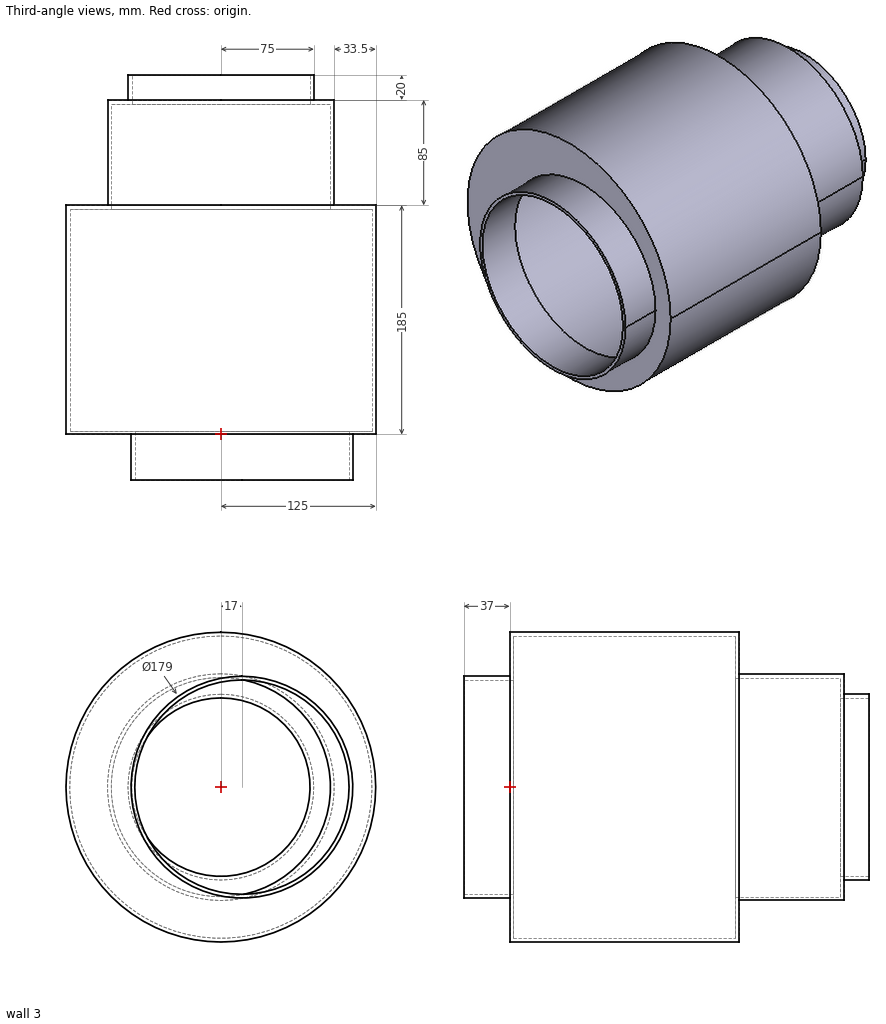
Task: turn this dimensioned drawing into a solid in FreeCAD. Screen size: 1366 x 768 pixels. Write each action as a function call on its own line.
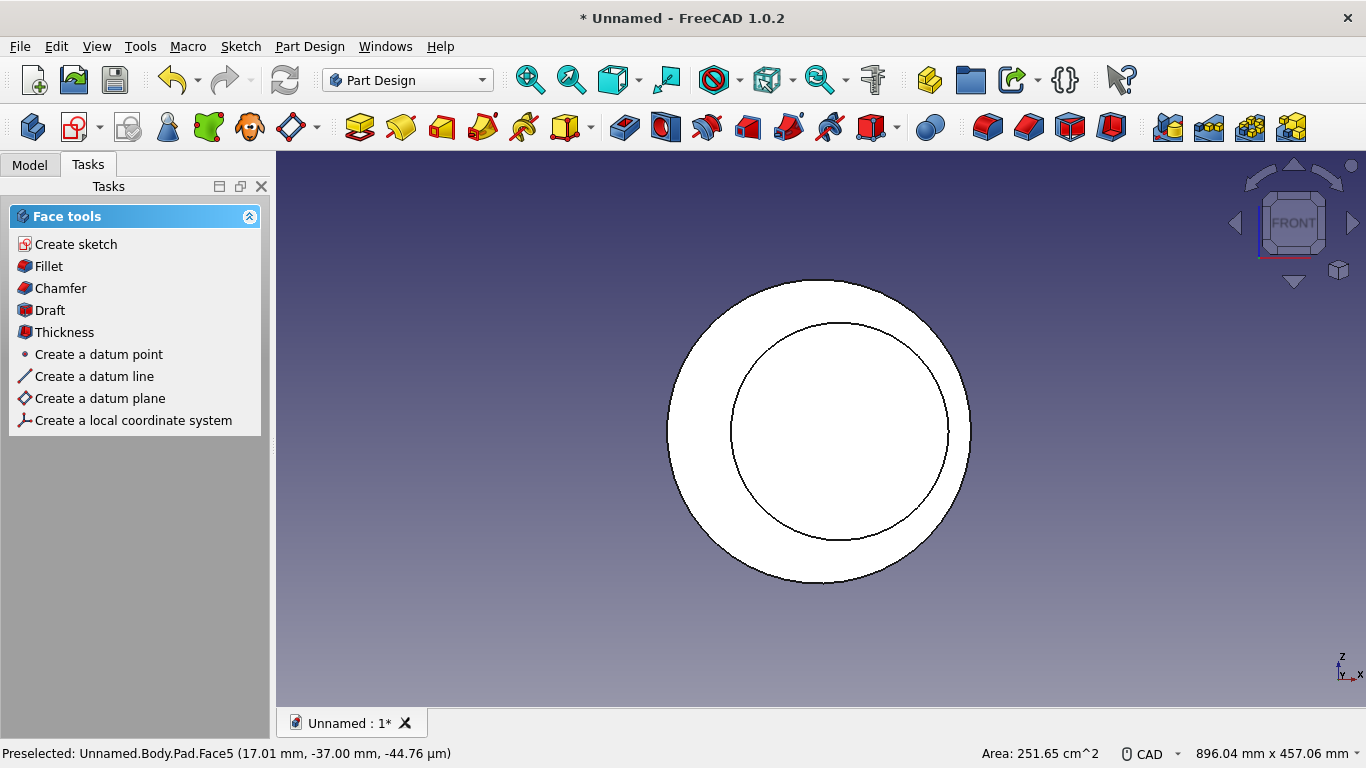
key(3)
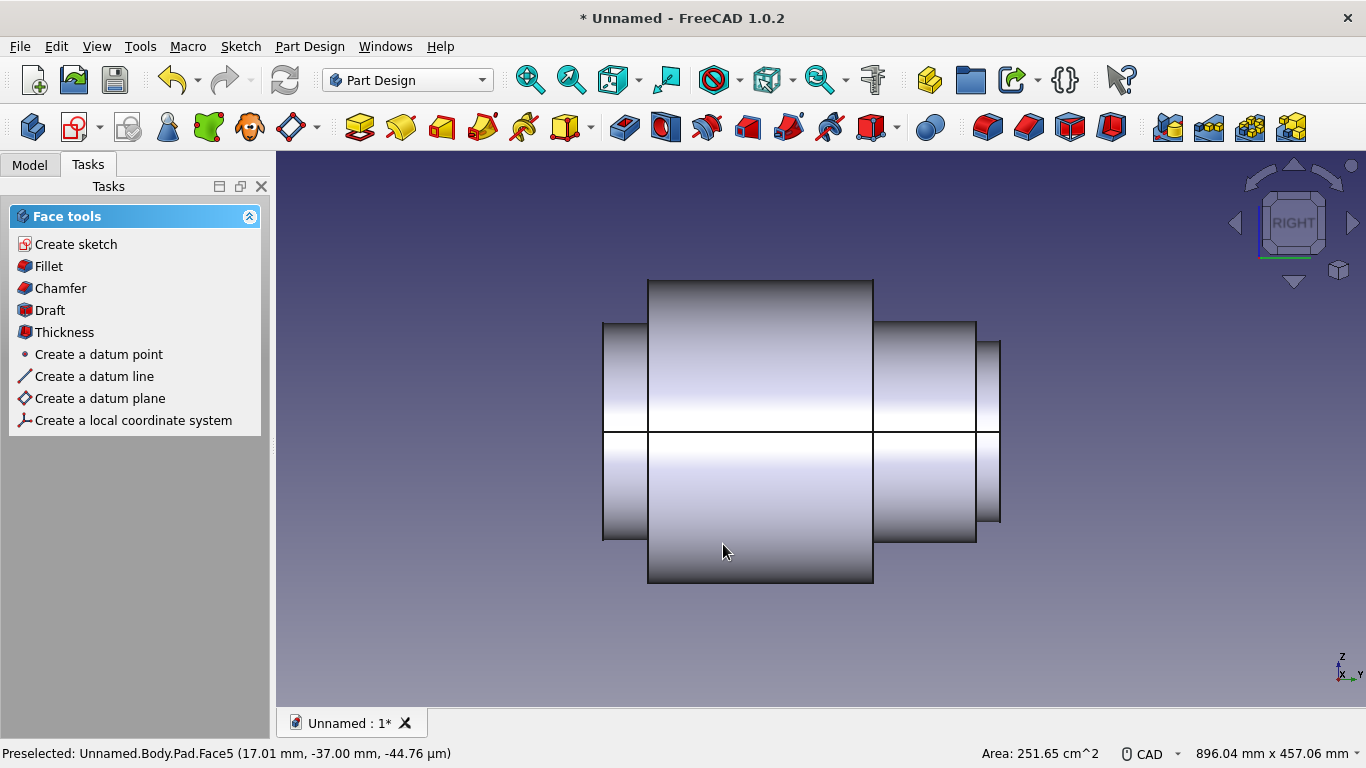
key(5)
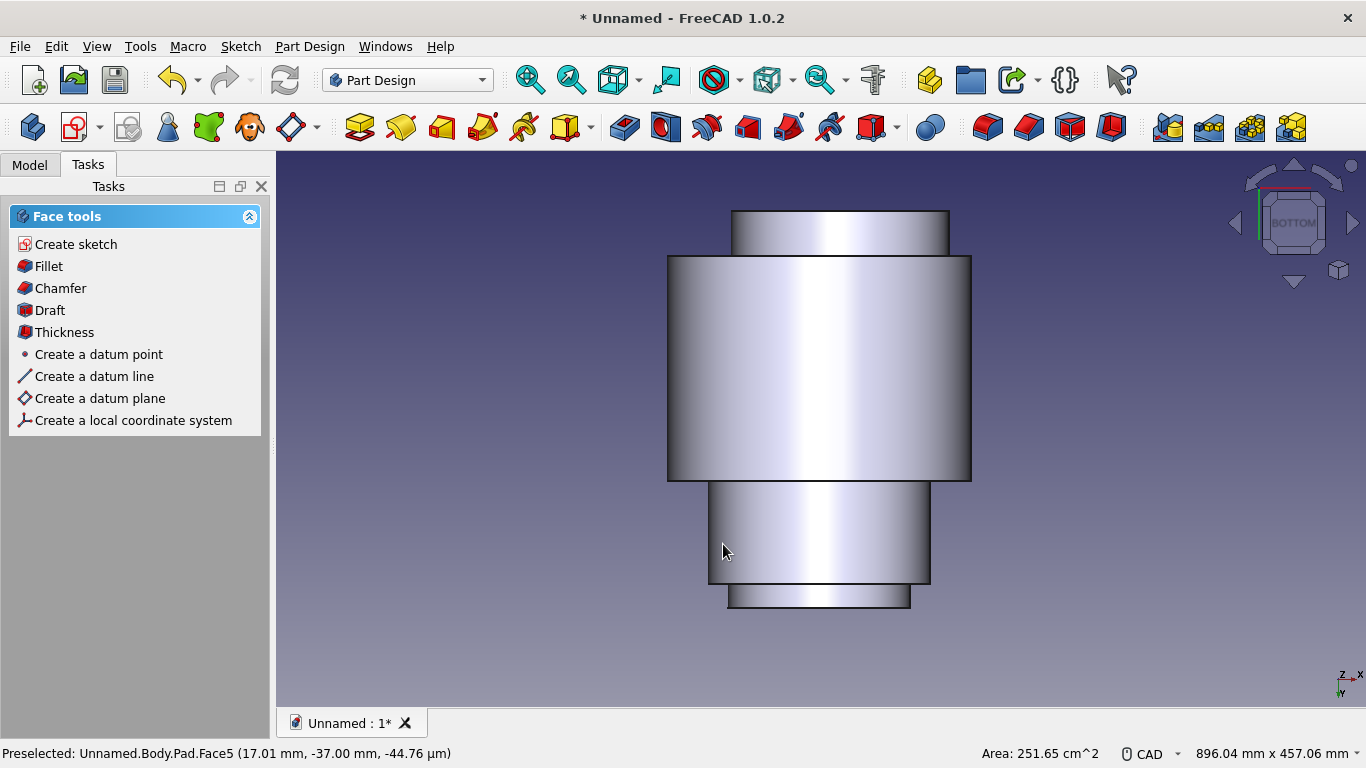
key(4)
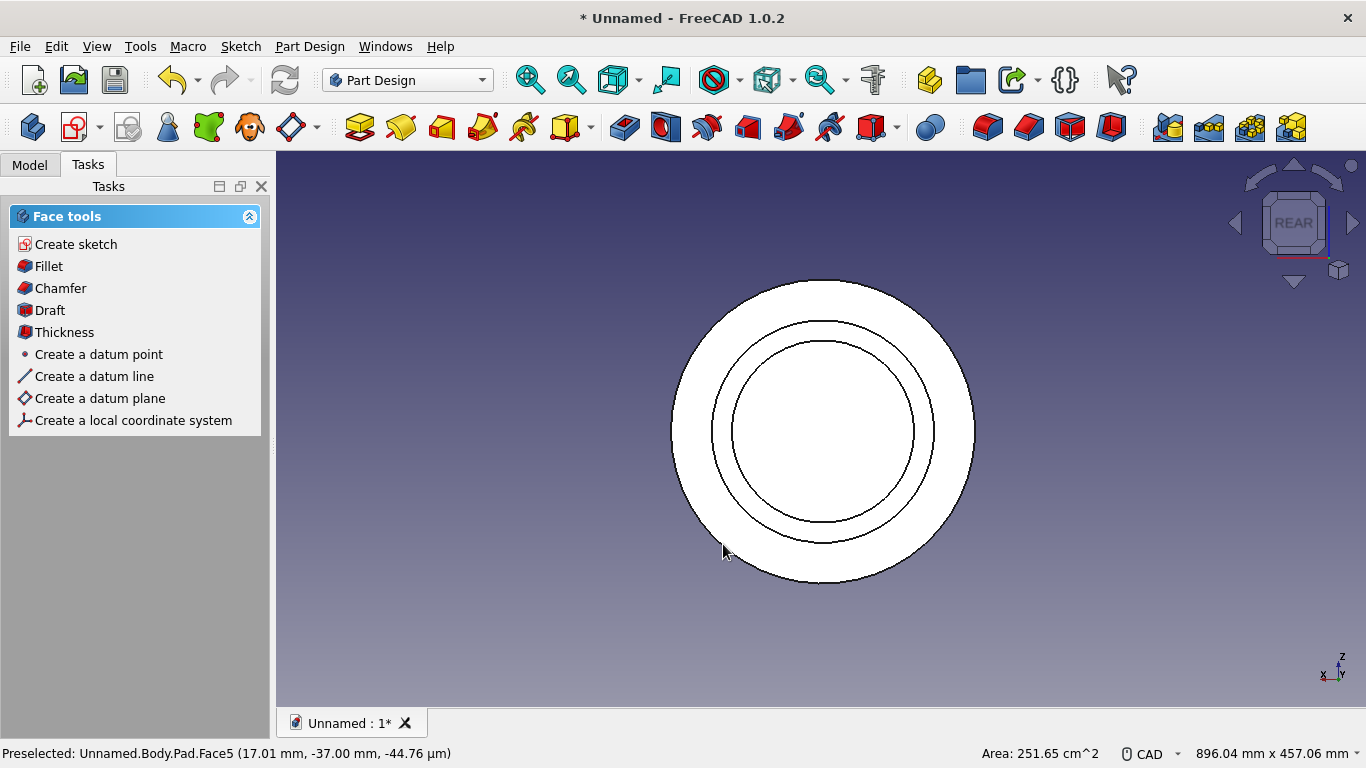
click(823, 431, ctrl)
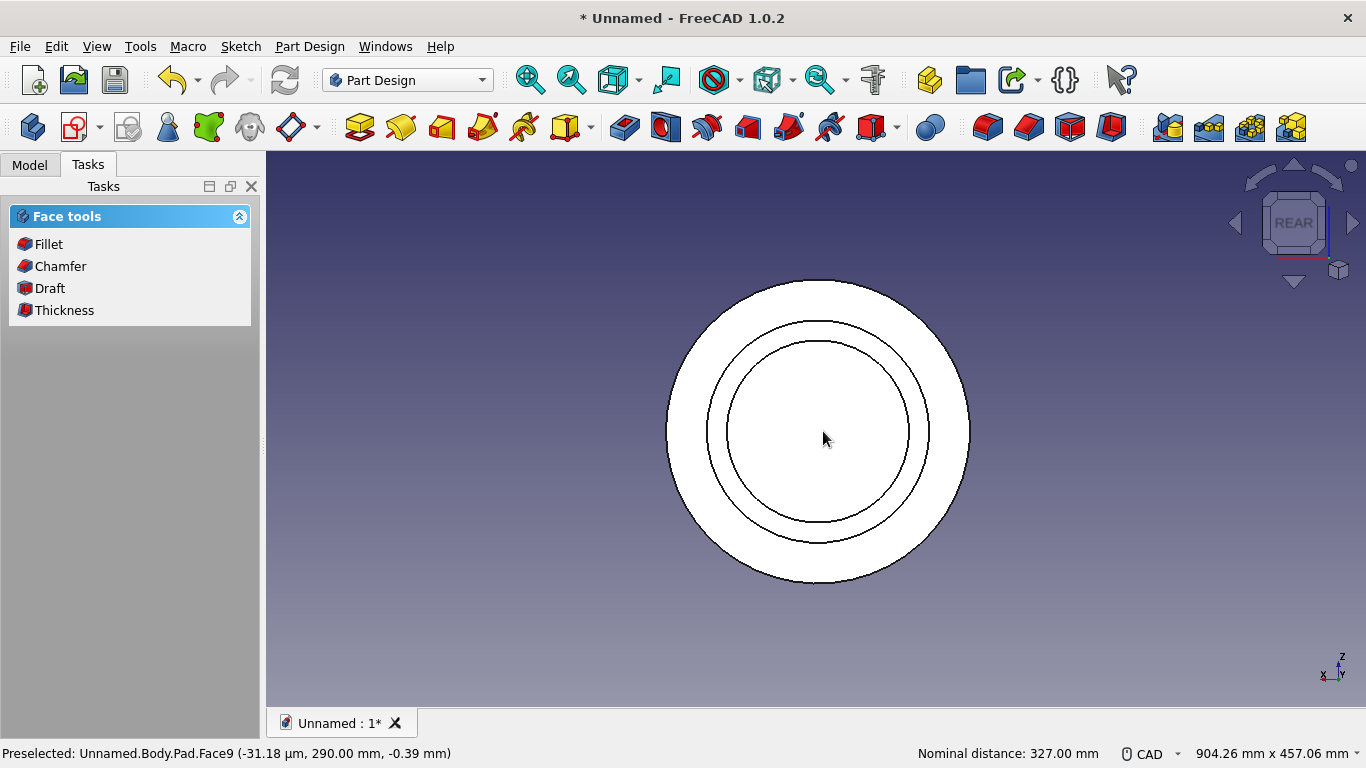
click(1111, 128)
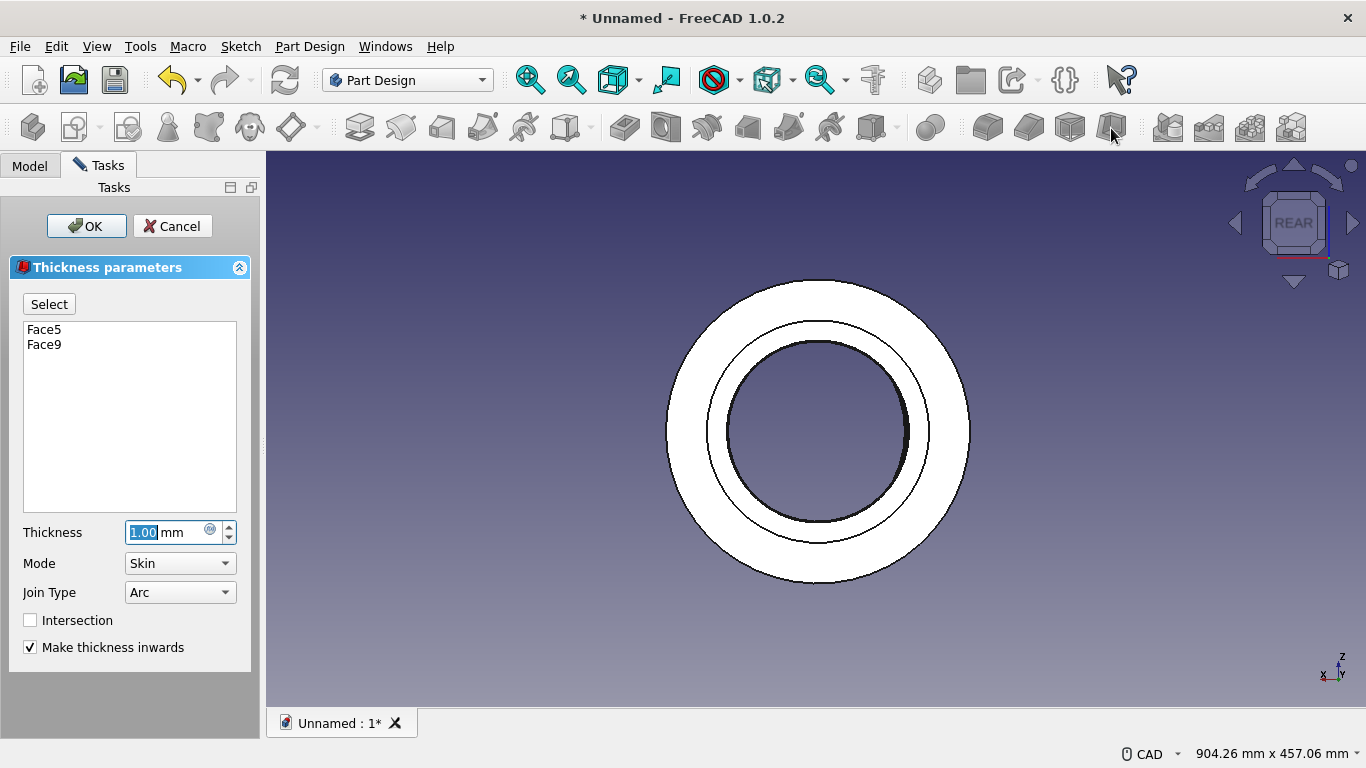
text(3)
key(Tab)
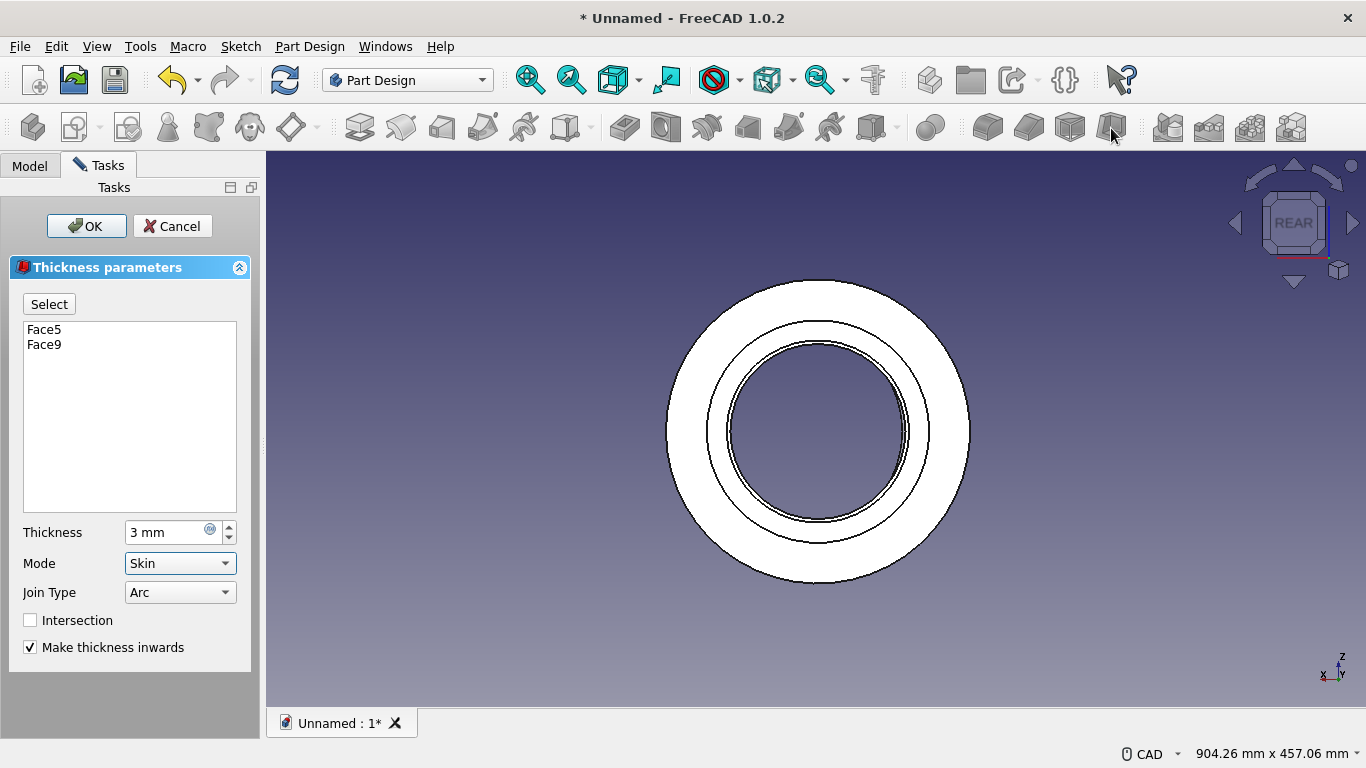
click(181, 592)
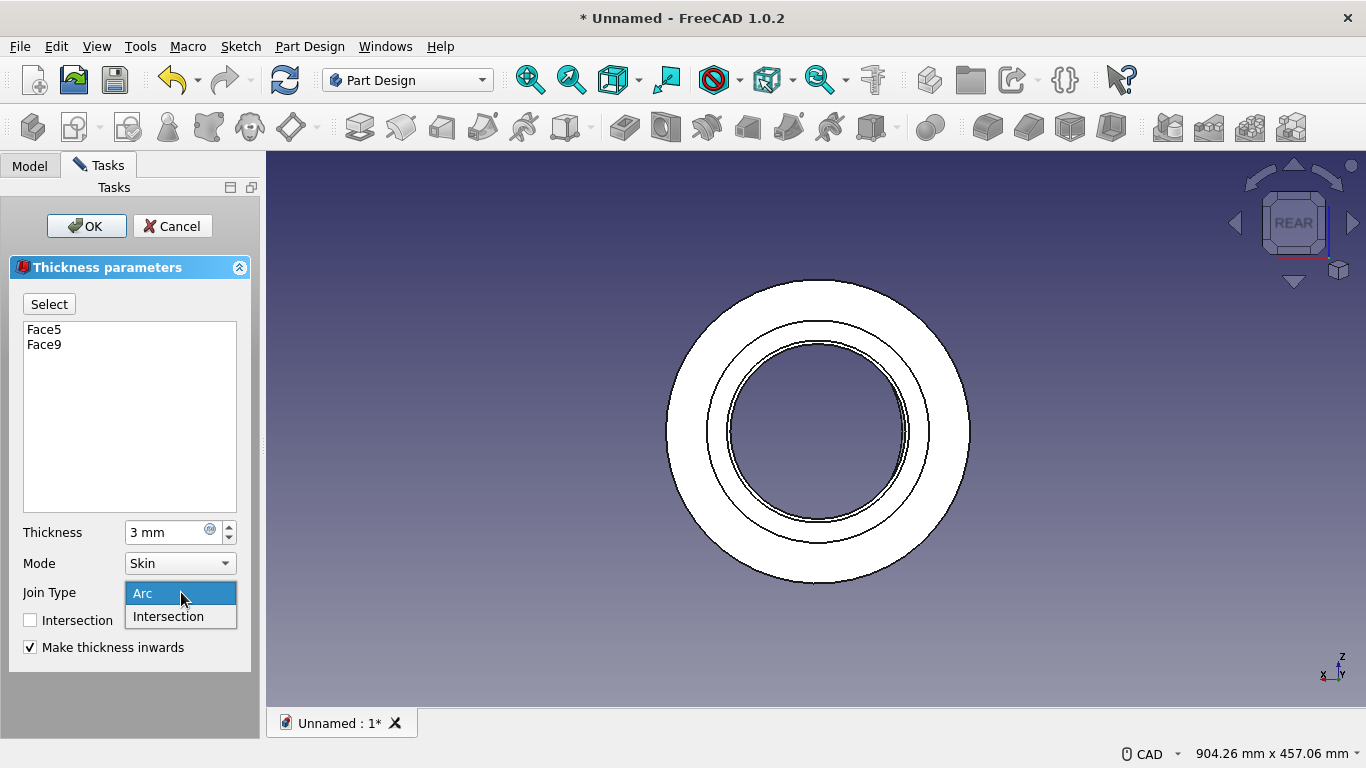
click(179, 616)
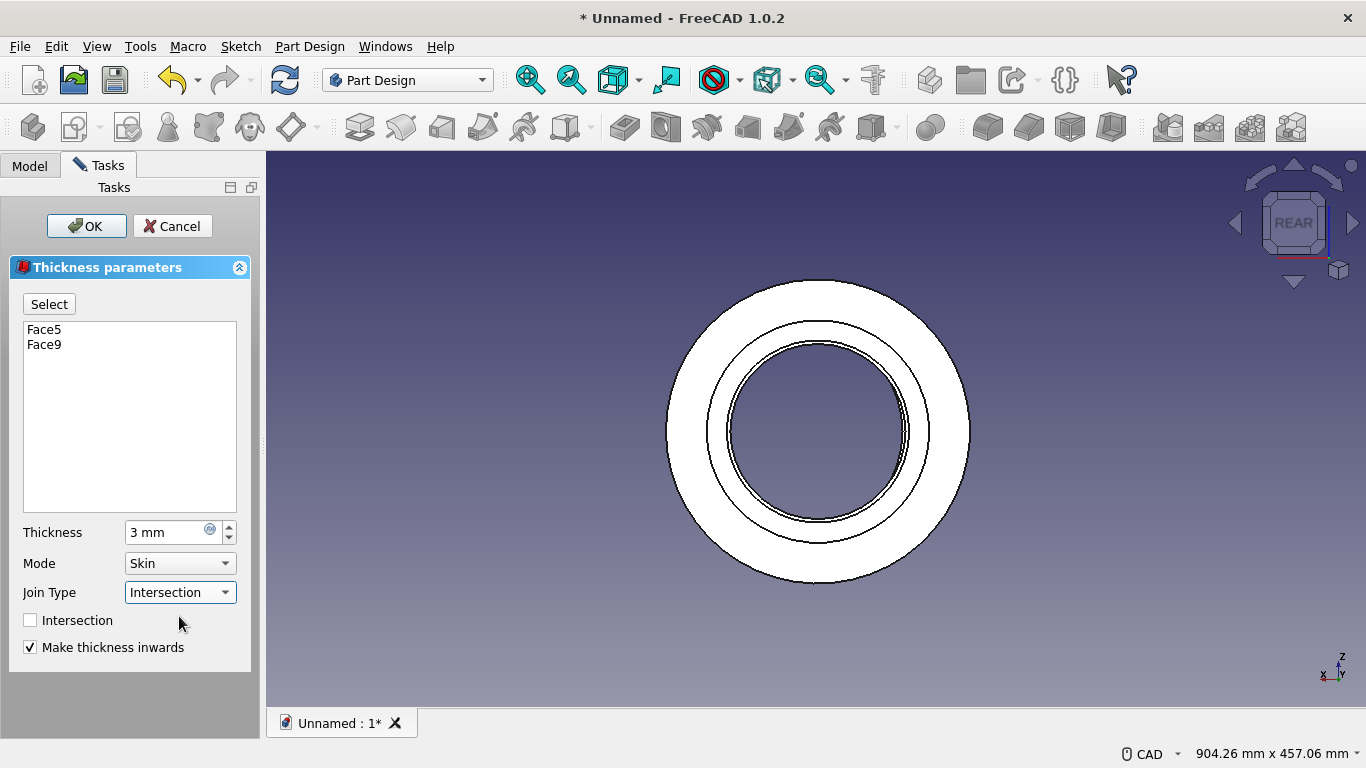
click(87, 226)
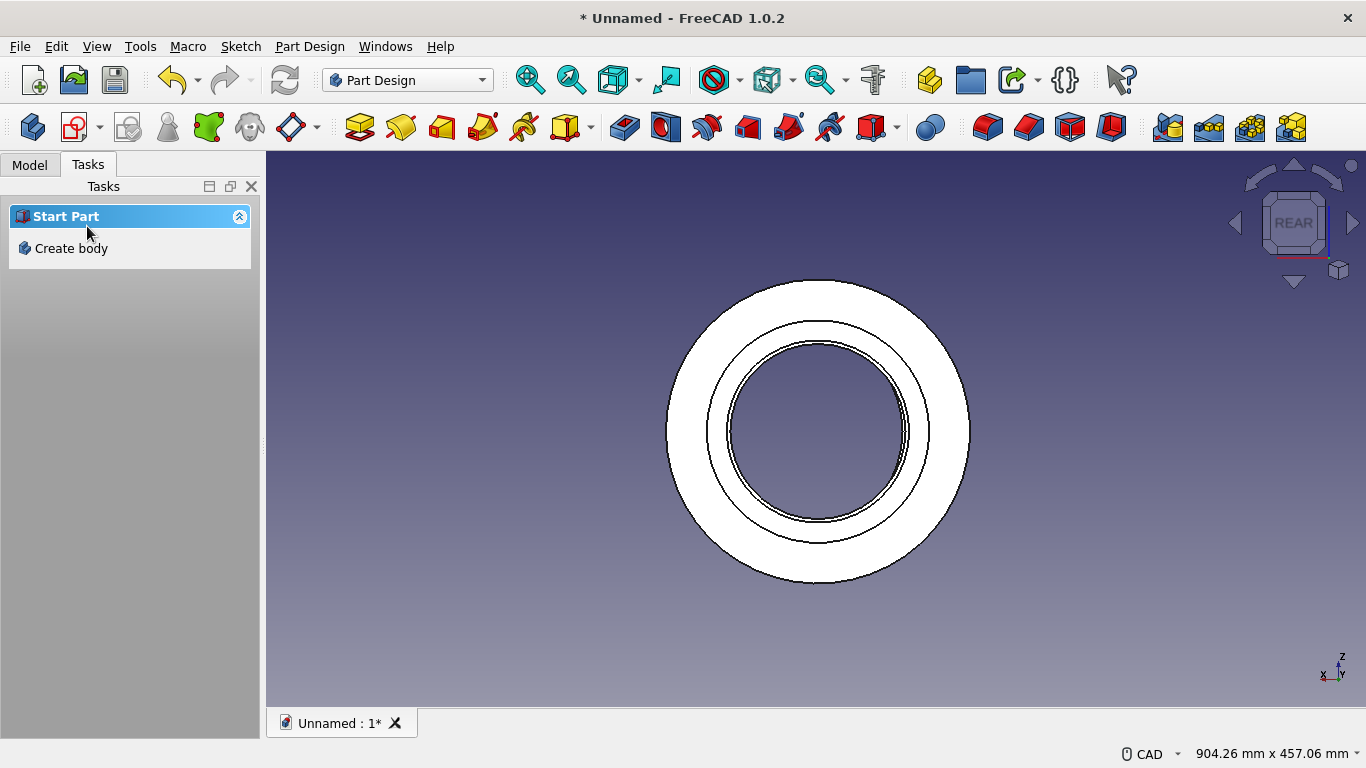
key(0)